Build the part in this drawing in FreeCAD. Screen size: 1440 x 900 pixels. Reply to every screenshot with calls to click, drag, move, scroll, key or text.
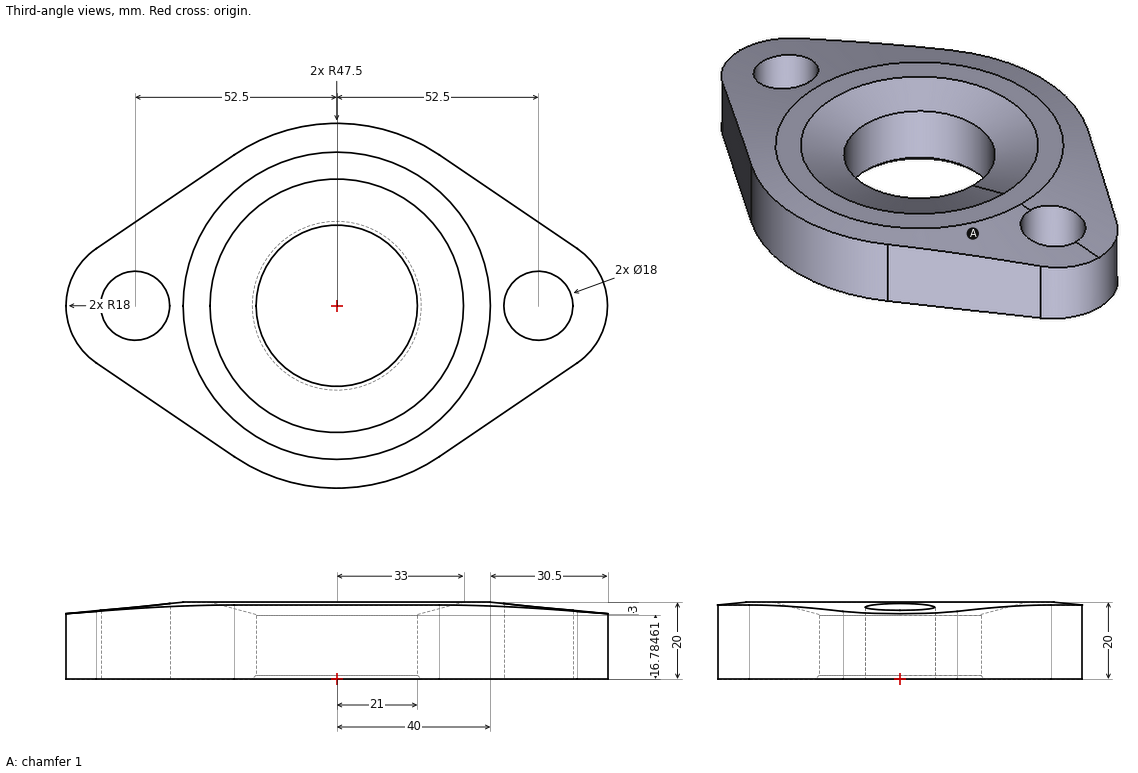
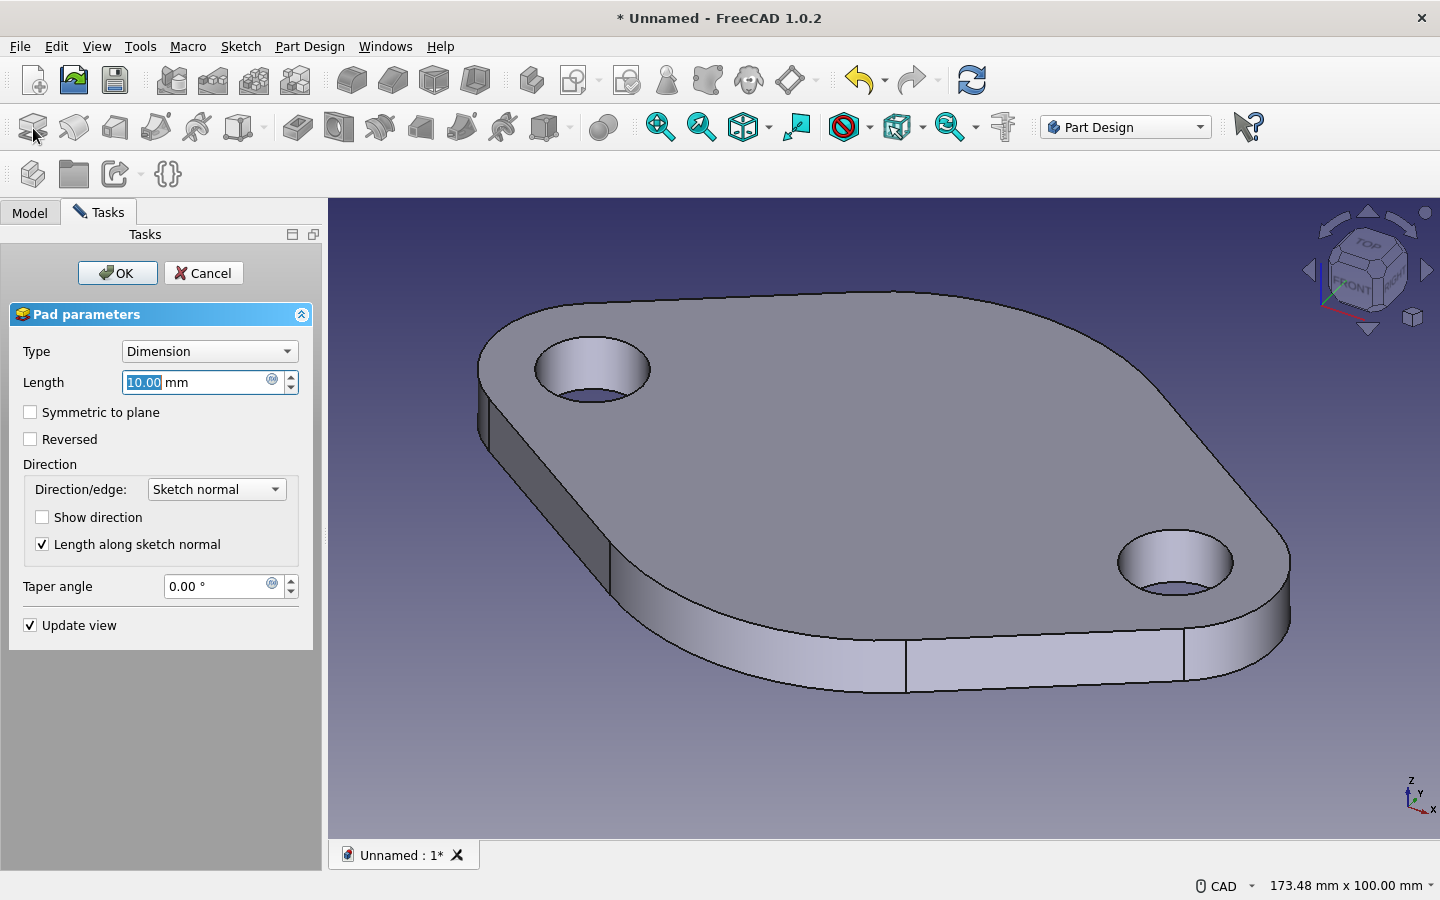
text(20)
key(Tab)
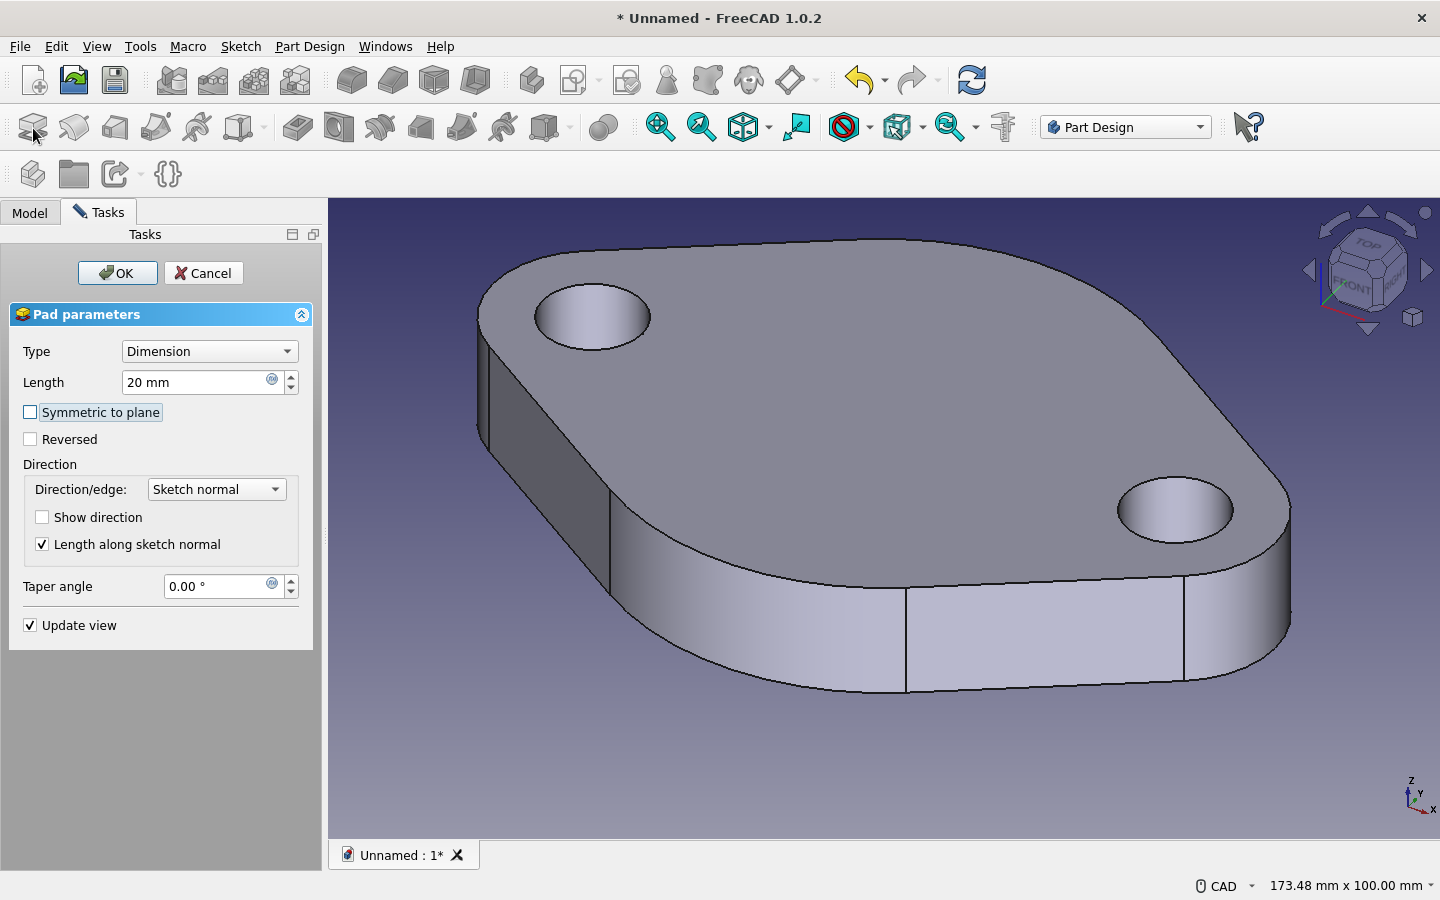
click(118, 273)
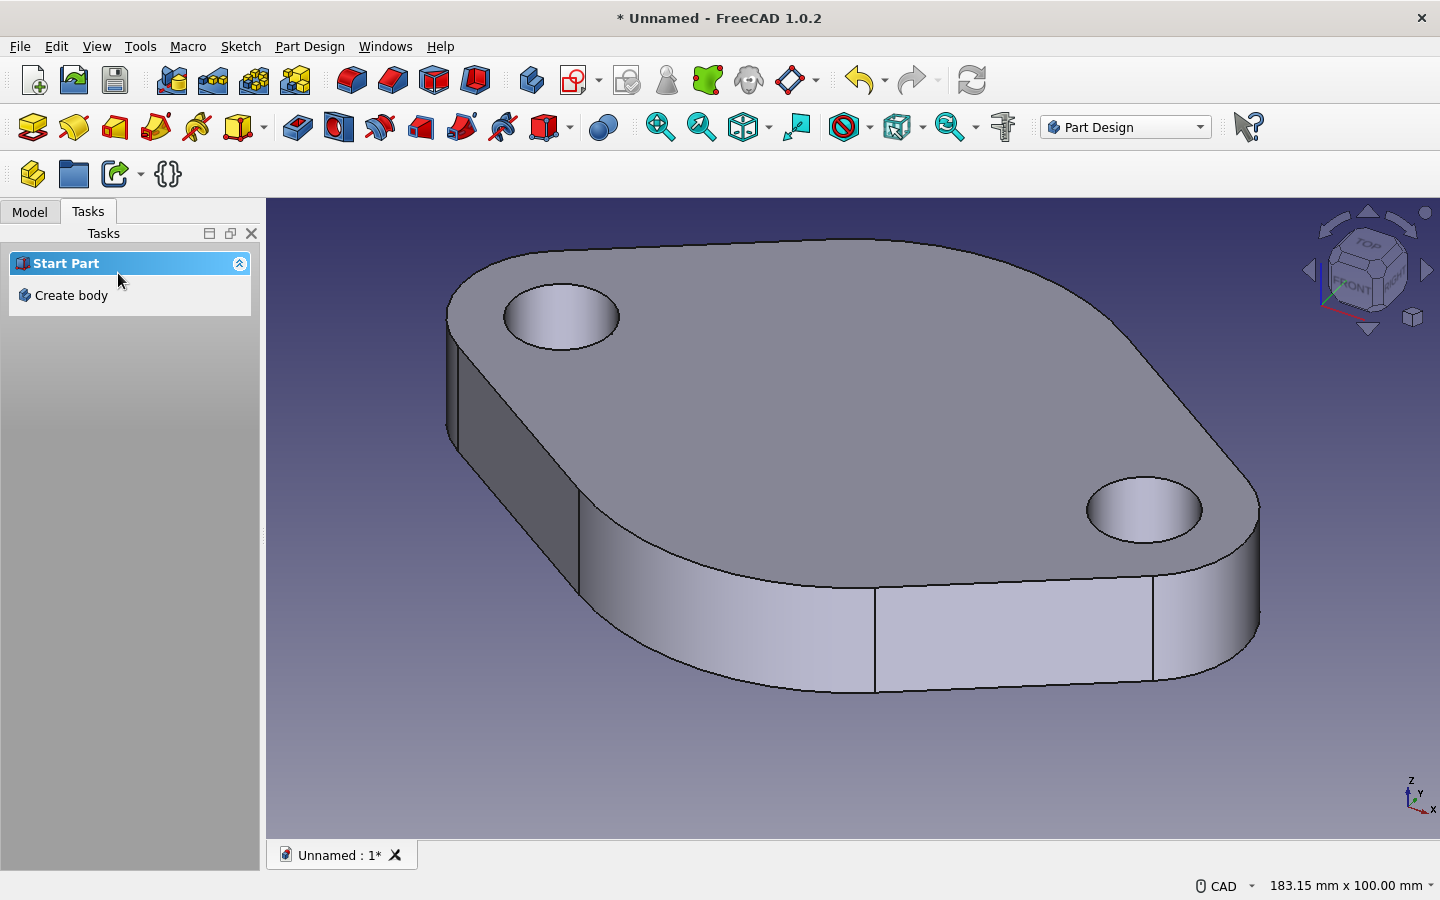
key(v)
key(f)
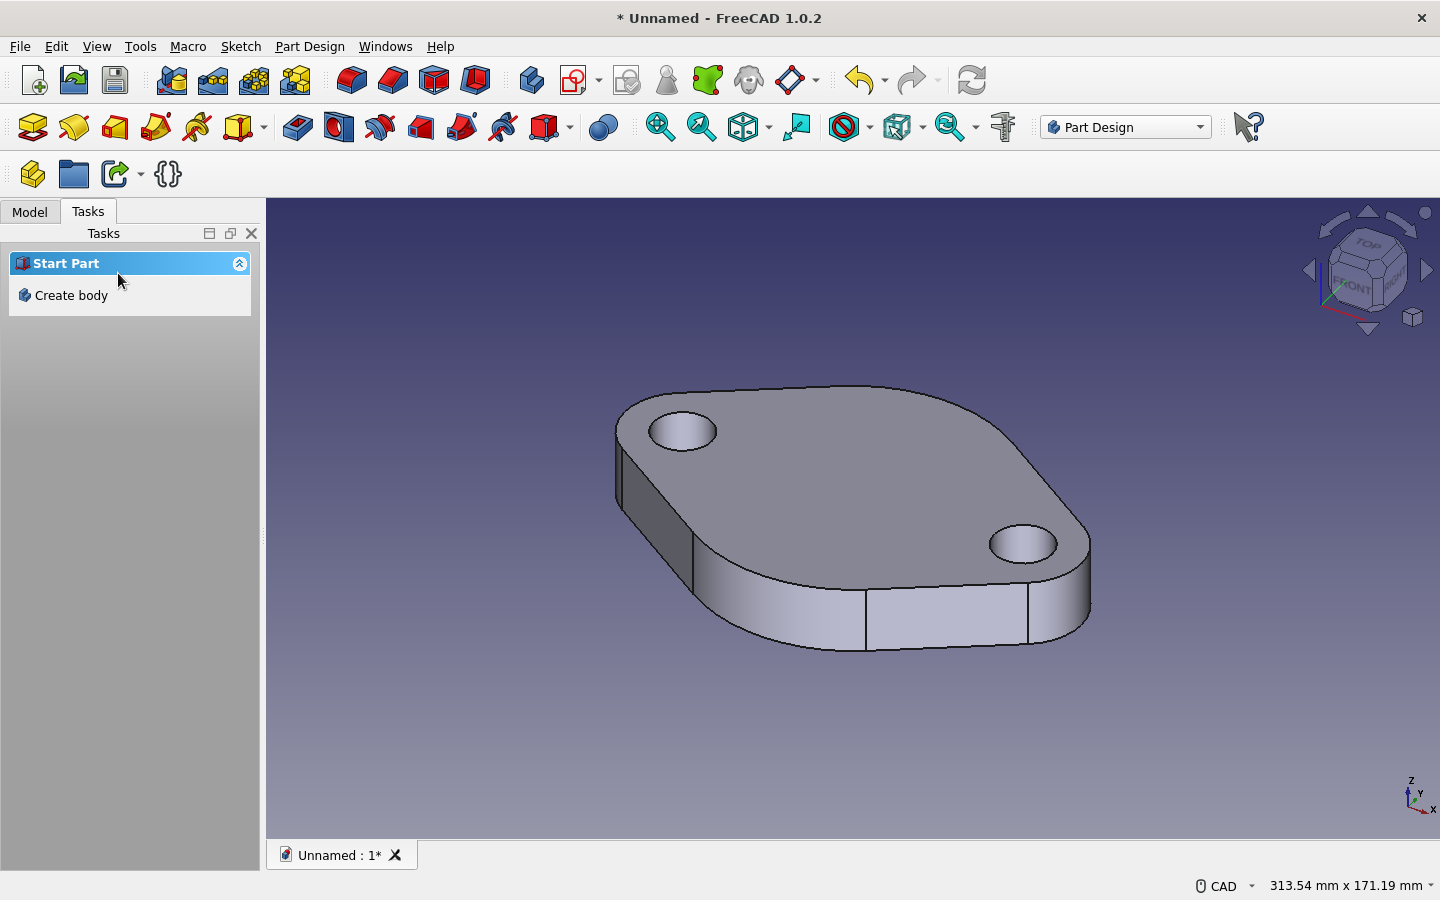
click(572, 80)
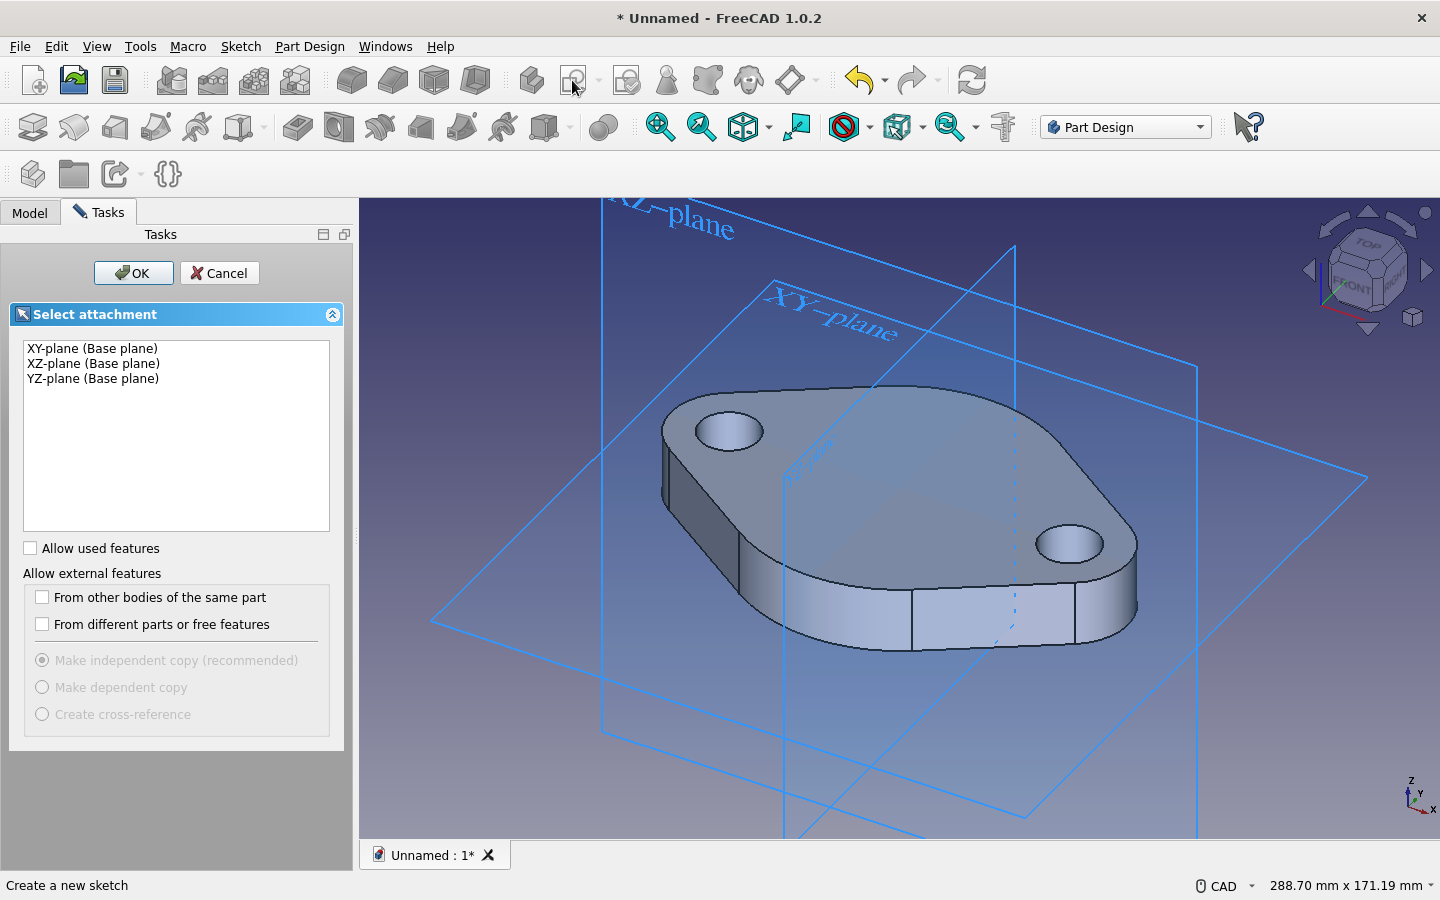
click(84, 364)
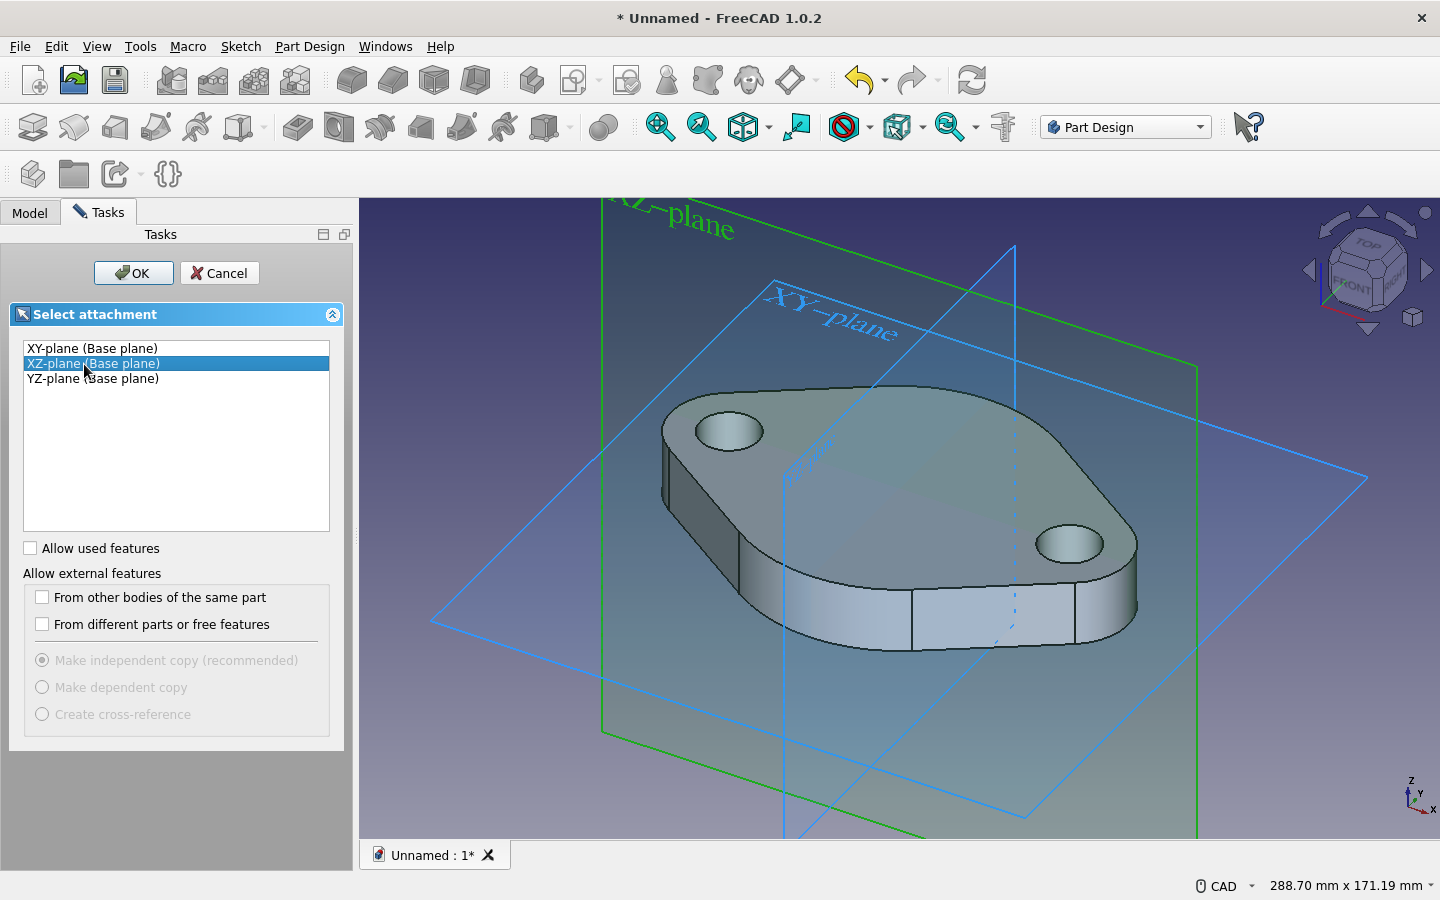
click(134, 273)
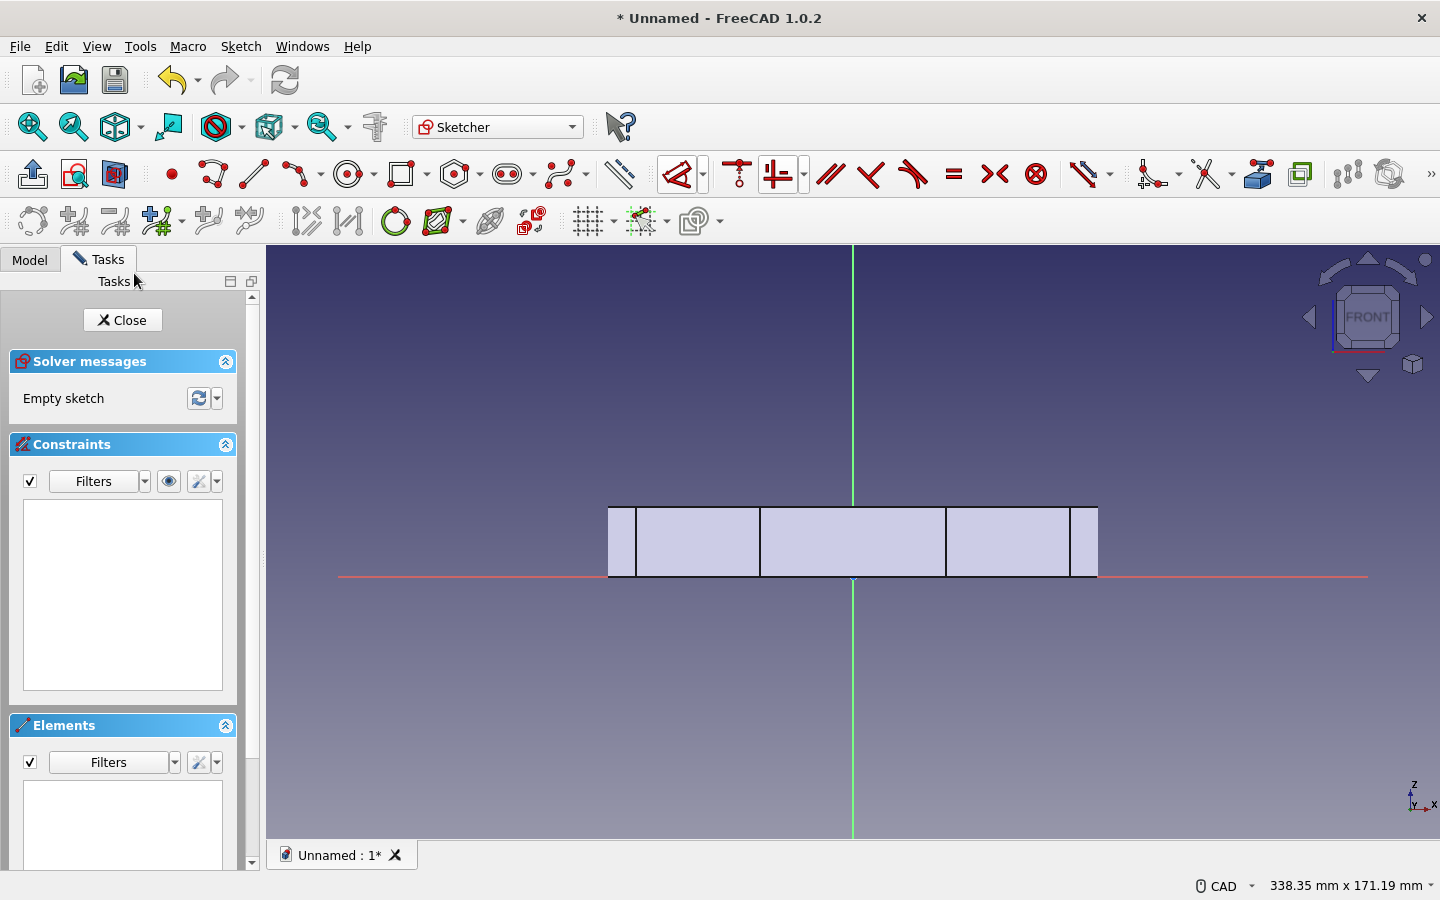
key(q)
key(s)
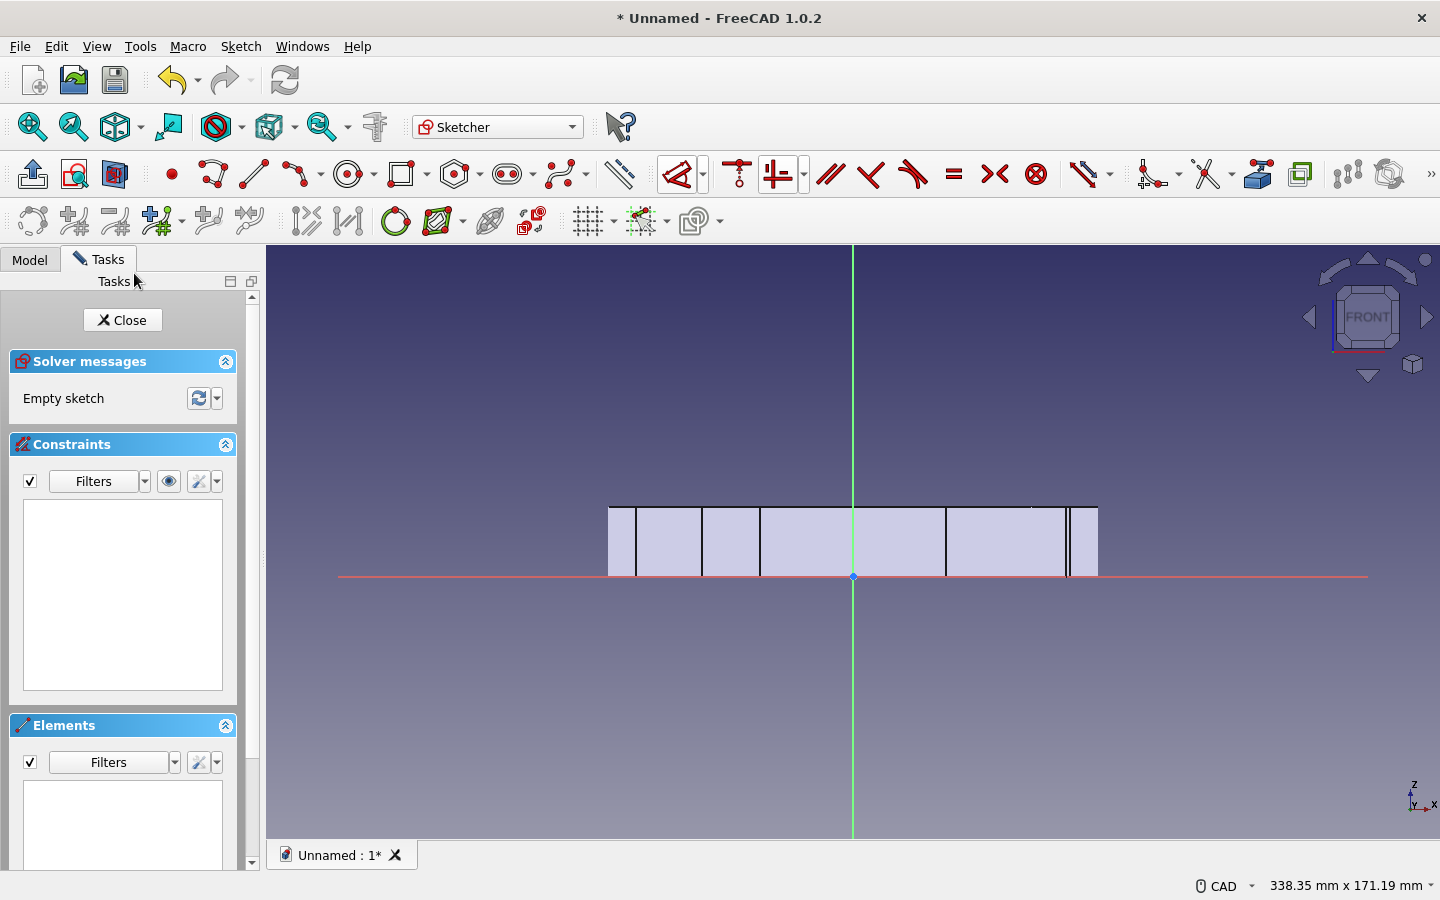
scroll(1086, 542, up, 5)